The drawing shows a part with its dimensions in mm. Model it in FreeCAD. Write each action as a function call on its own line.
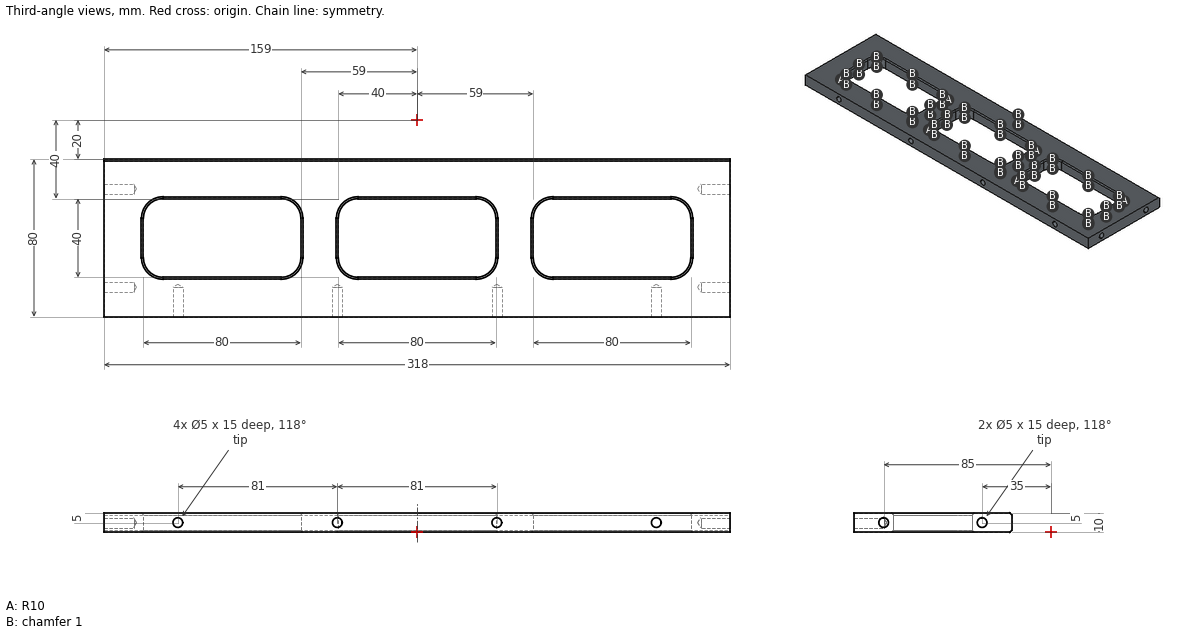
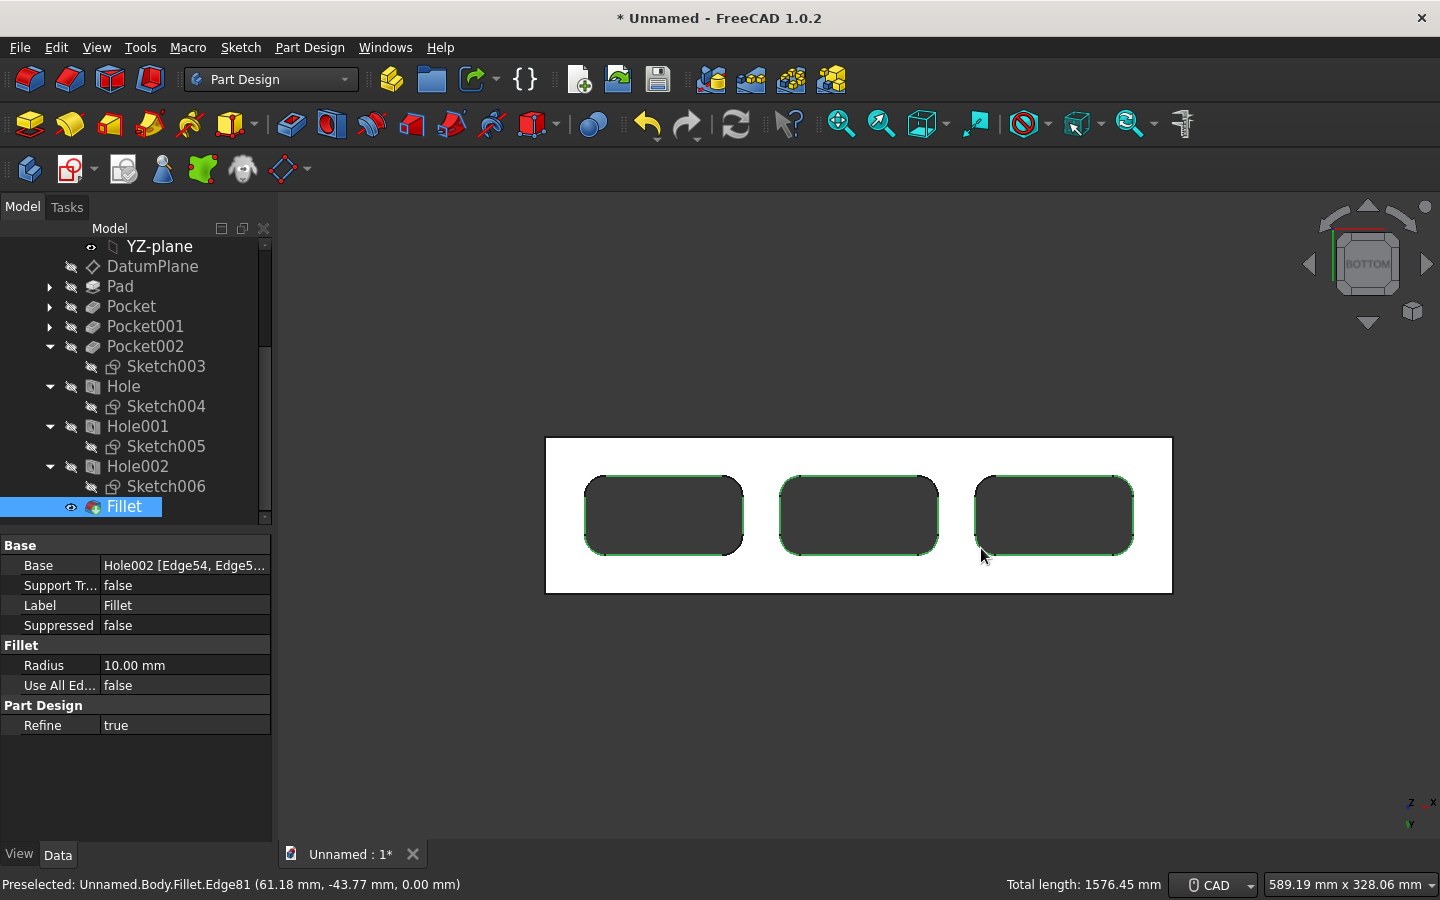
click(932, 481, ctrl)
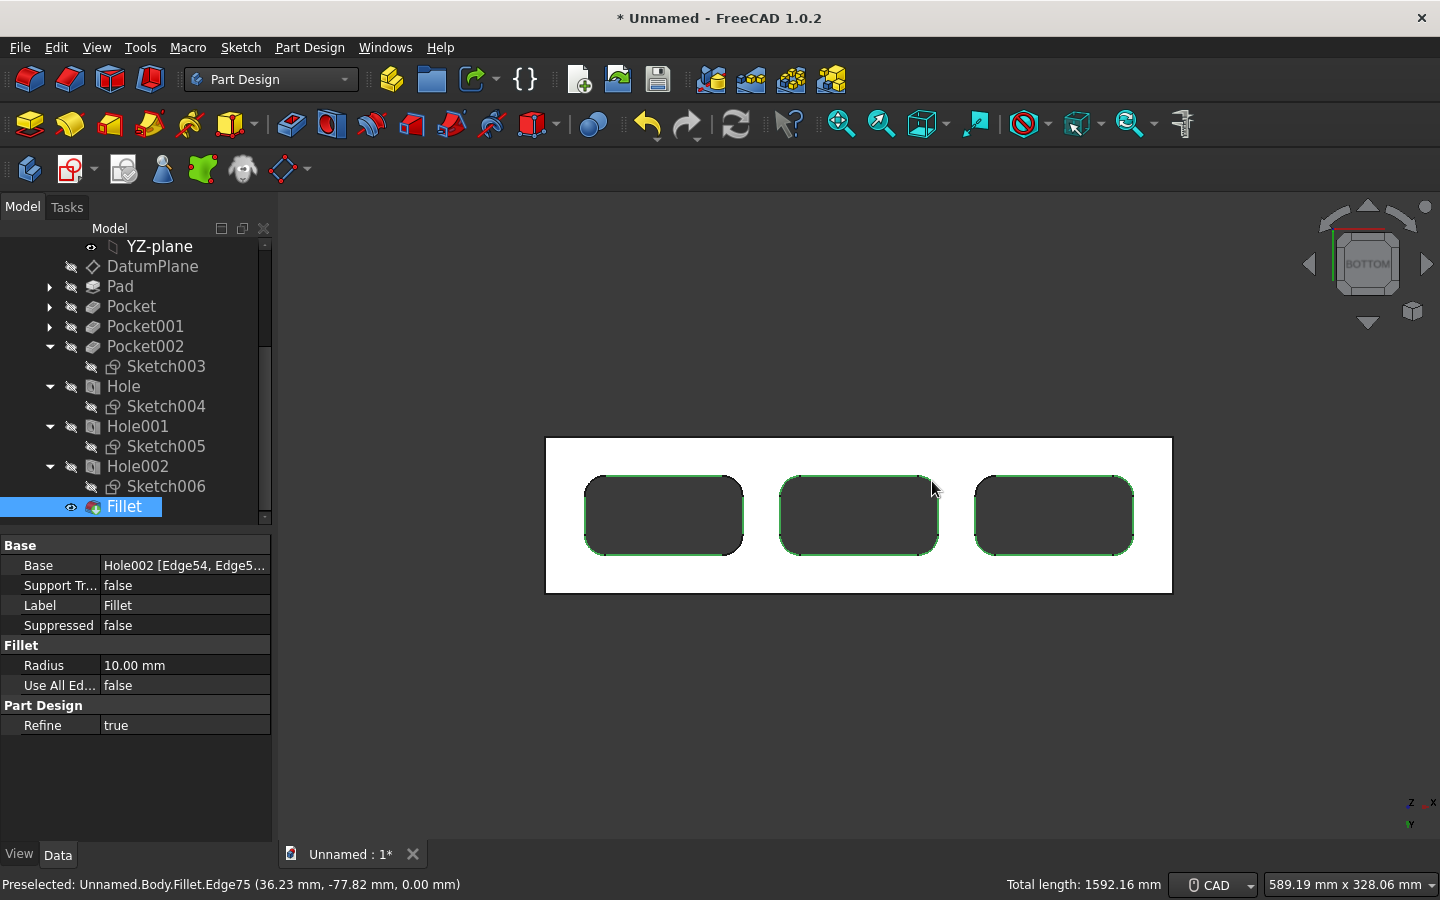
click(737, 548, ctrl)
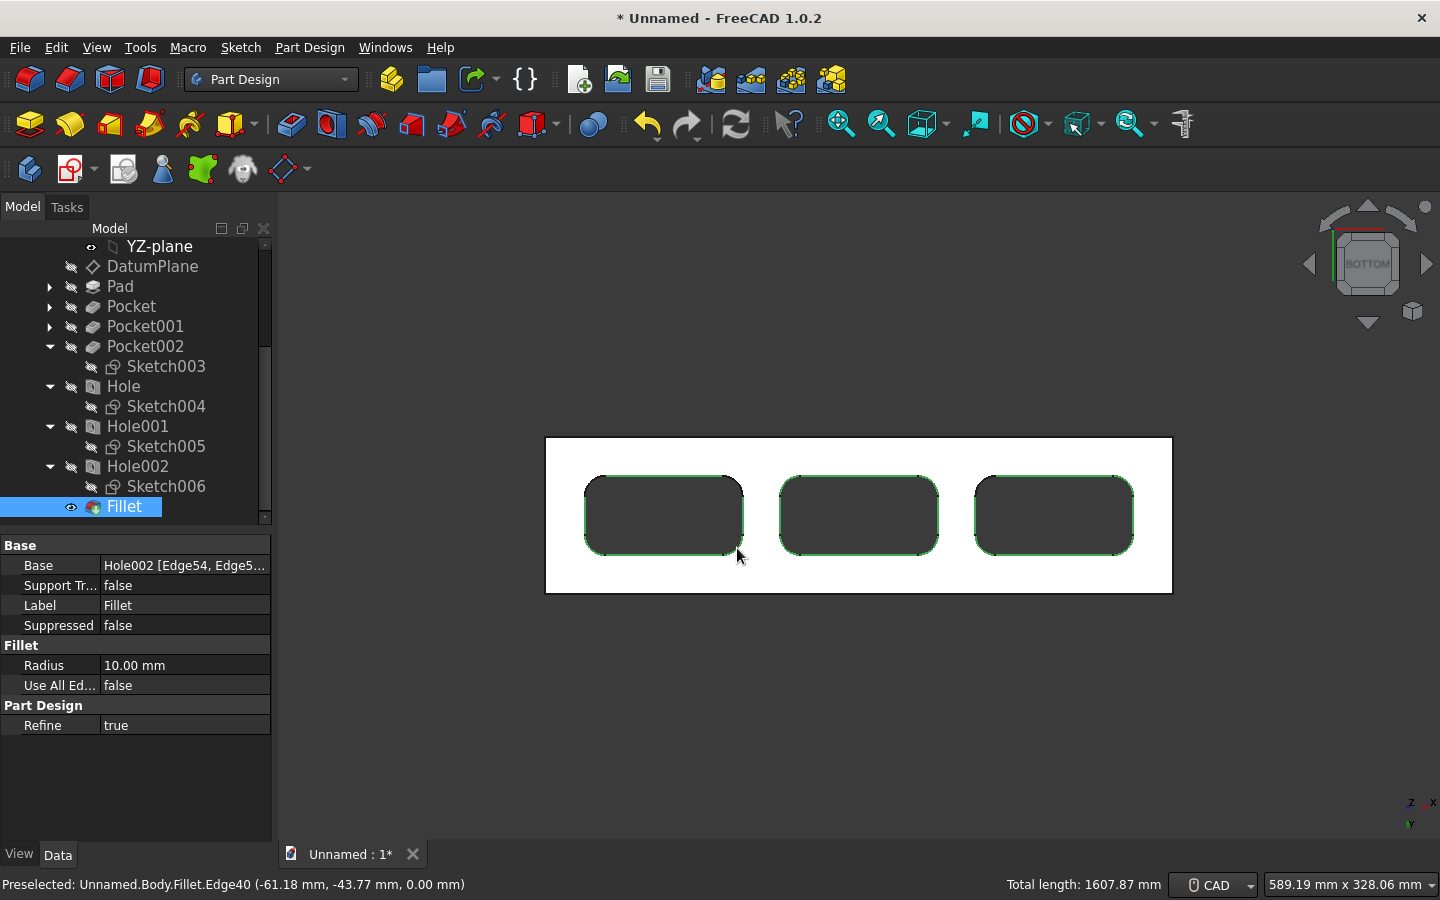
click(737, 481, ctrl)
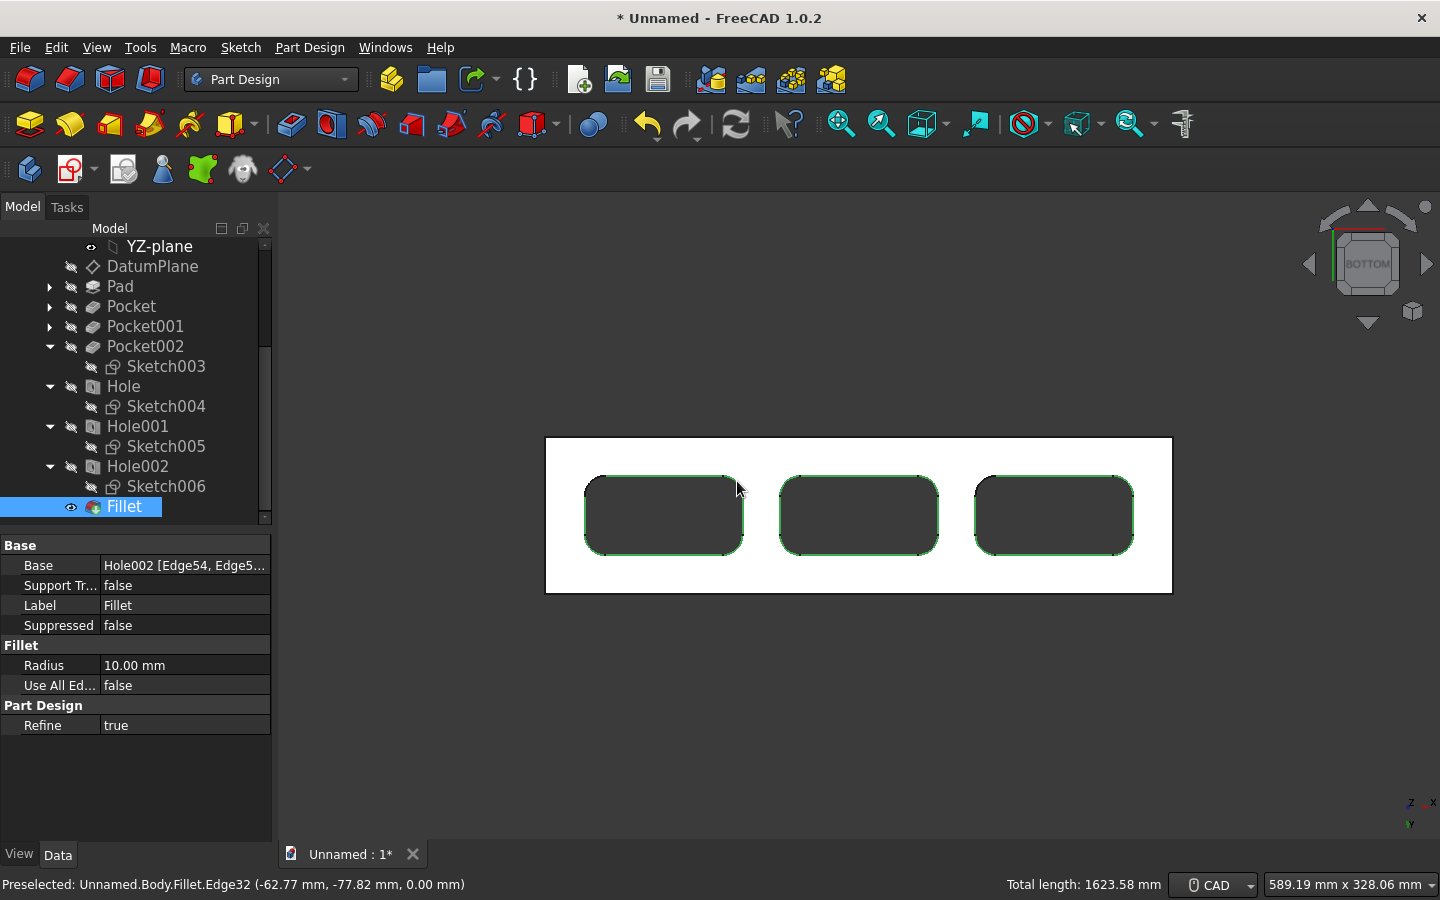
click(591, 481, ctrl)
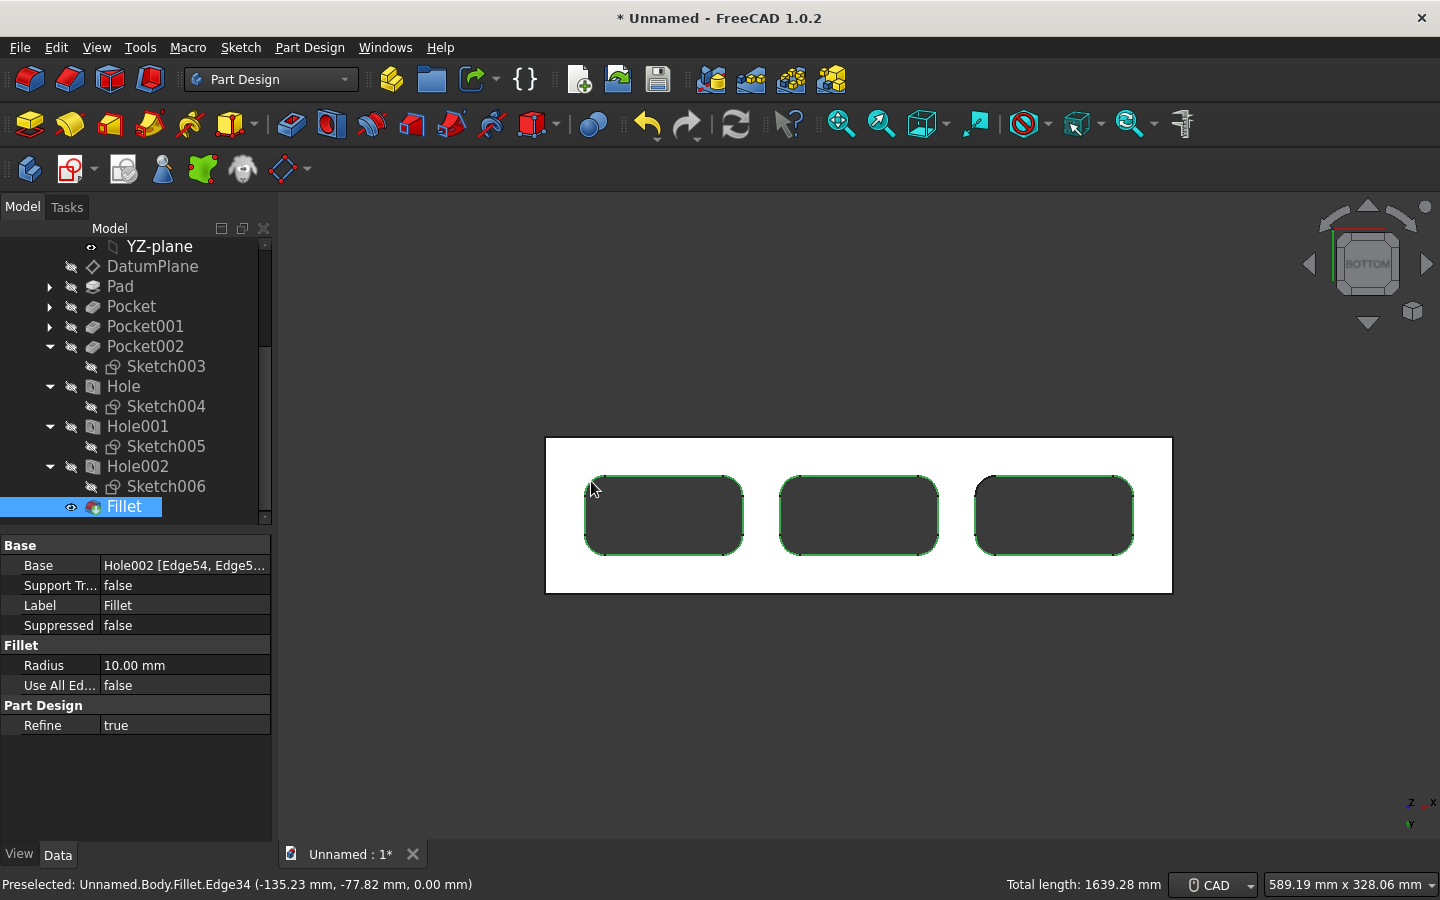
click(981, 481, ctrl)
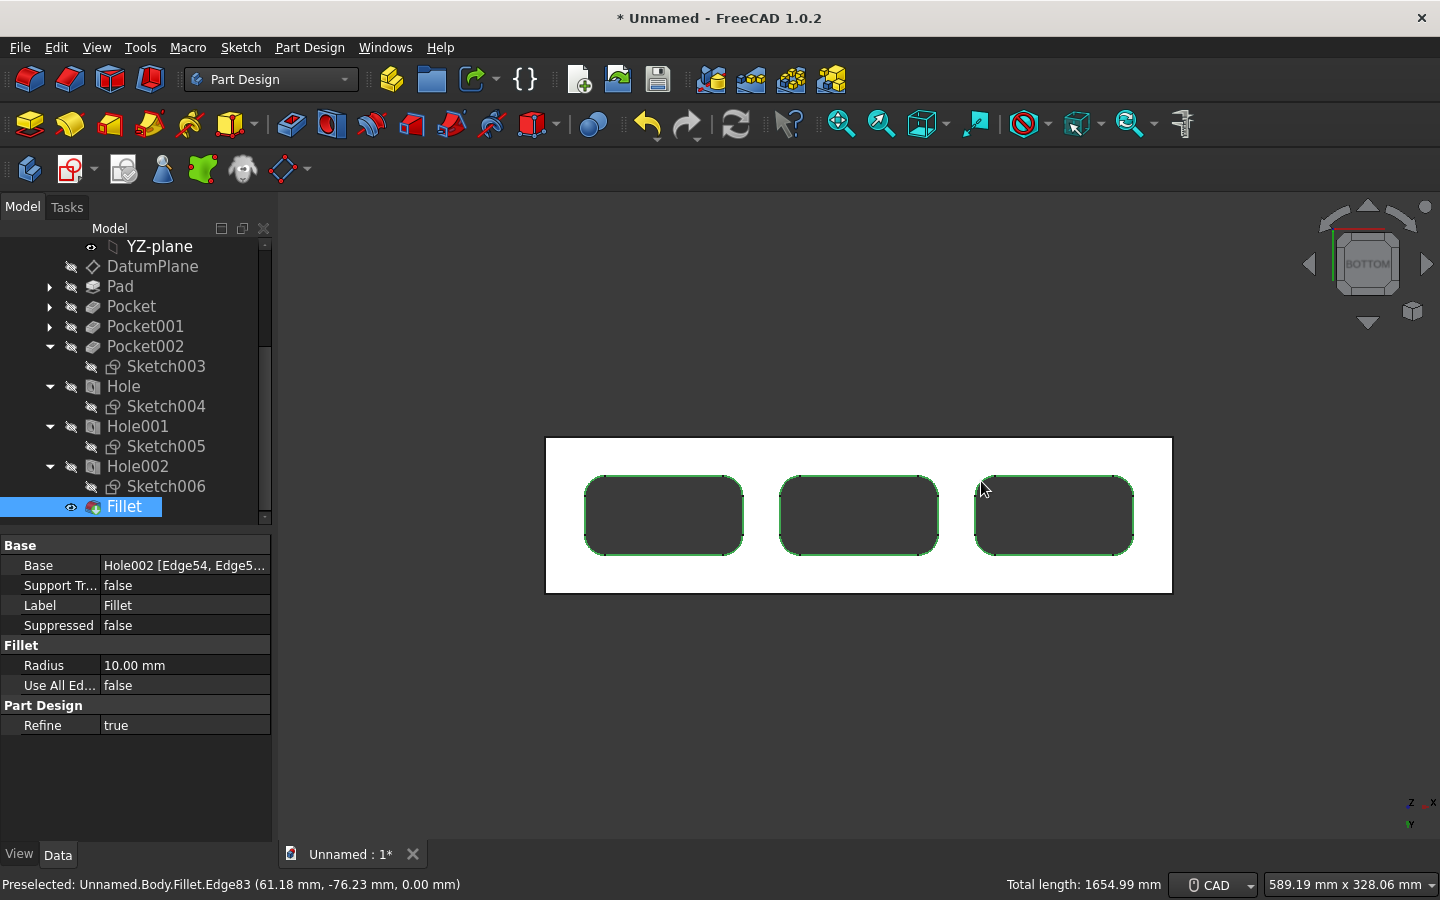
click(859, 593, ctrl)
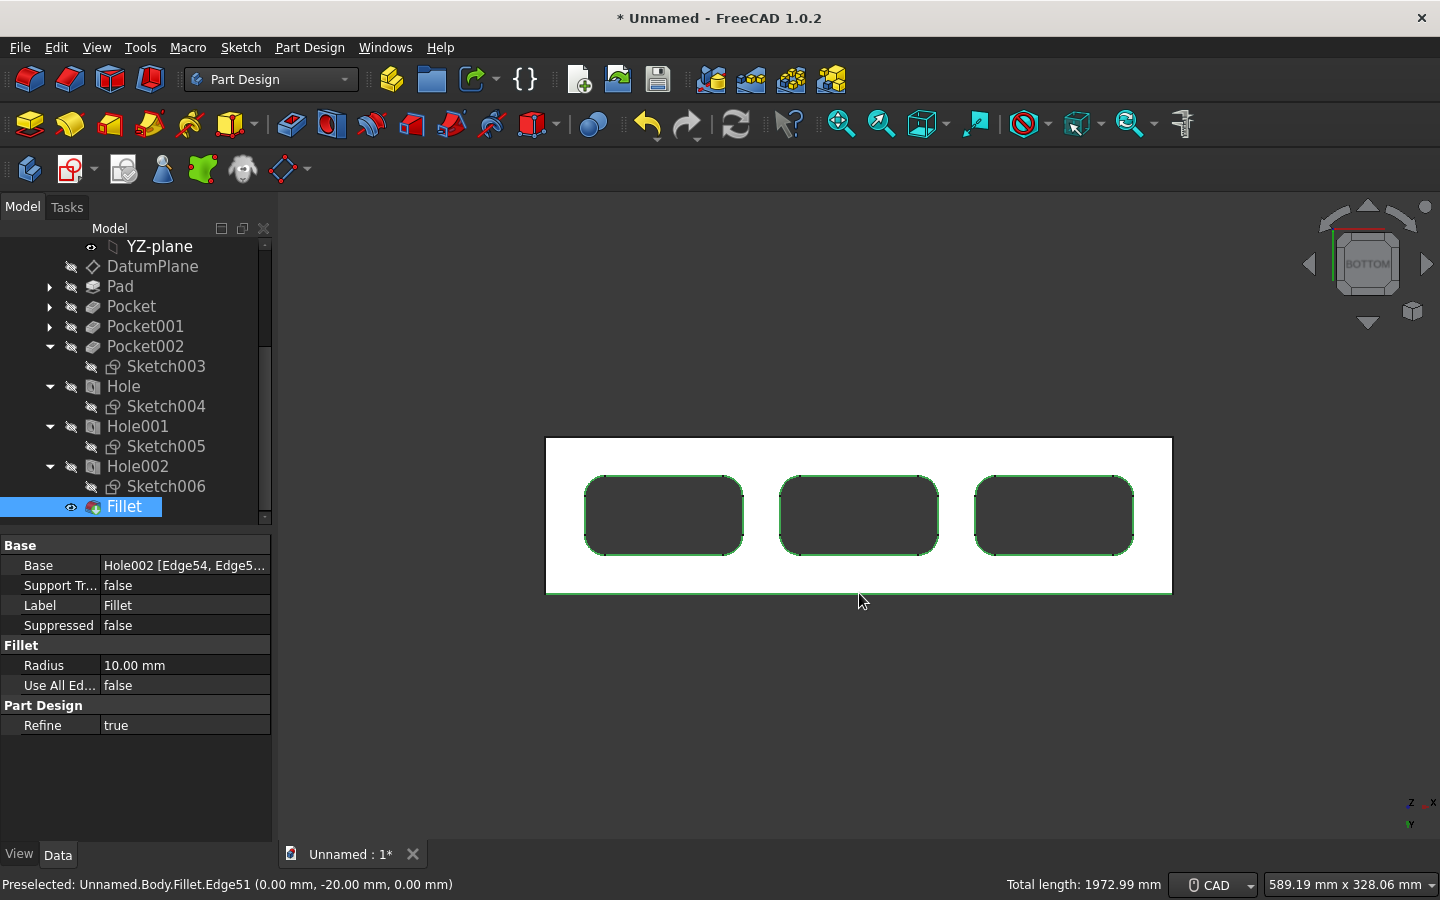
click(70, 80)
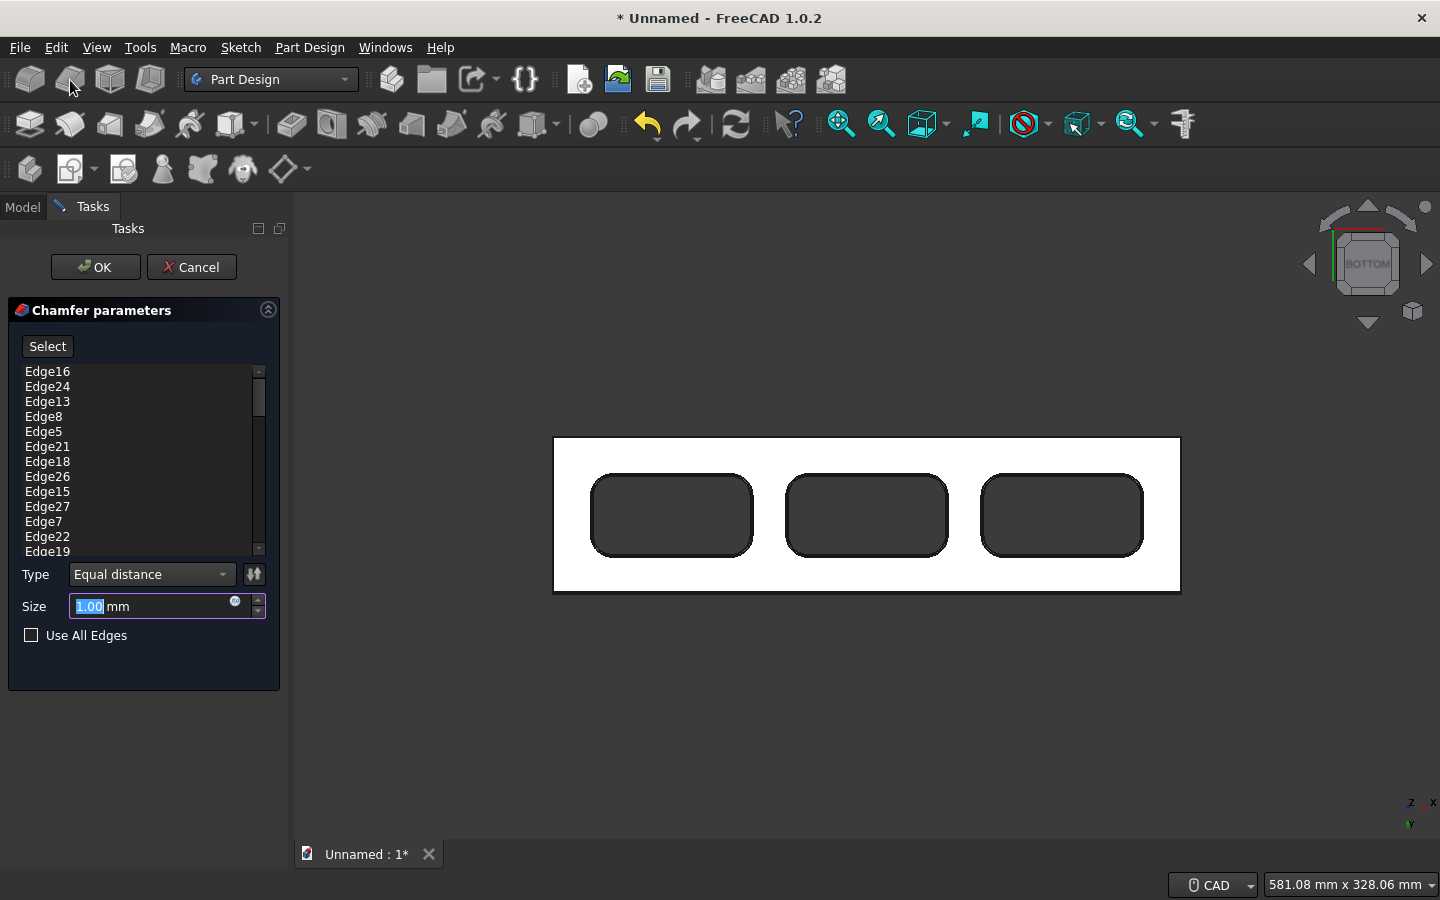
text(1)
key(Tab)